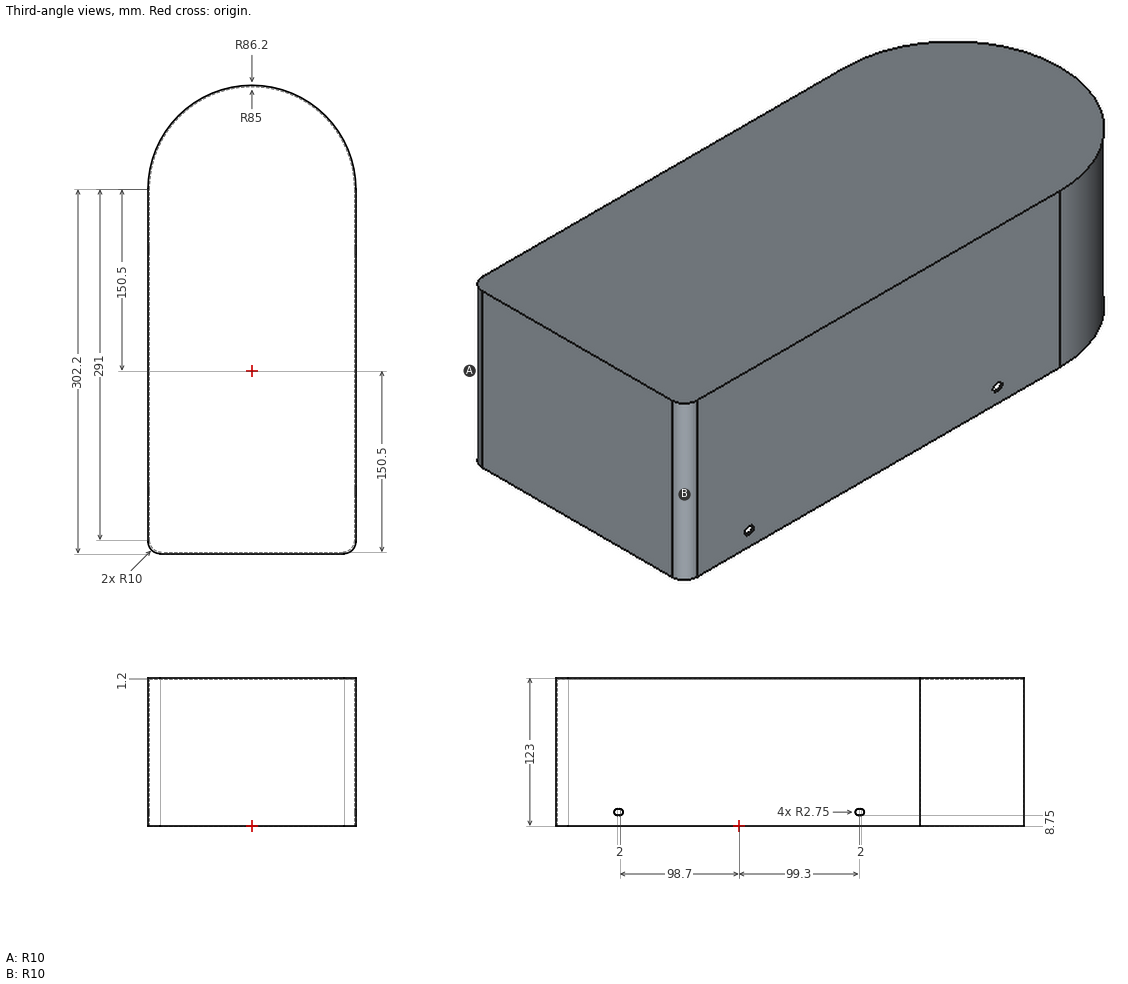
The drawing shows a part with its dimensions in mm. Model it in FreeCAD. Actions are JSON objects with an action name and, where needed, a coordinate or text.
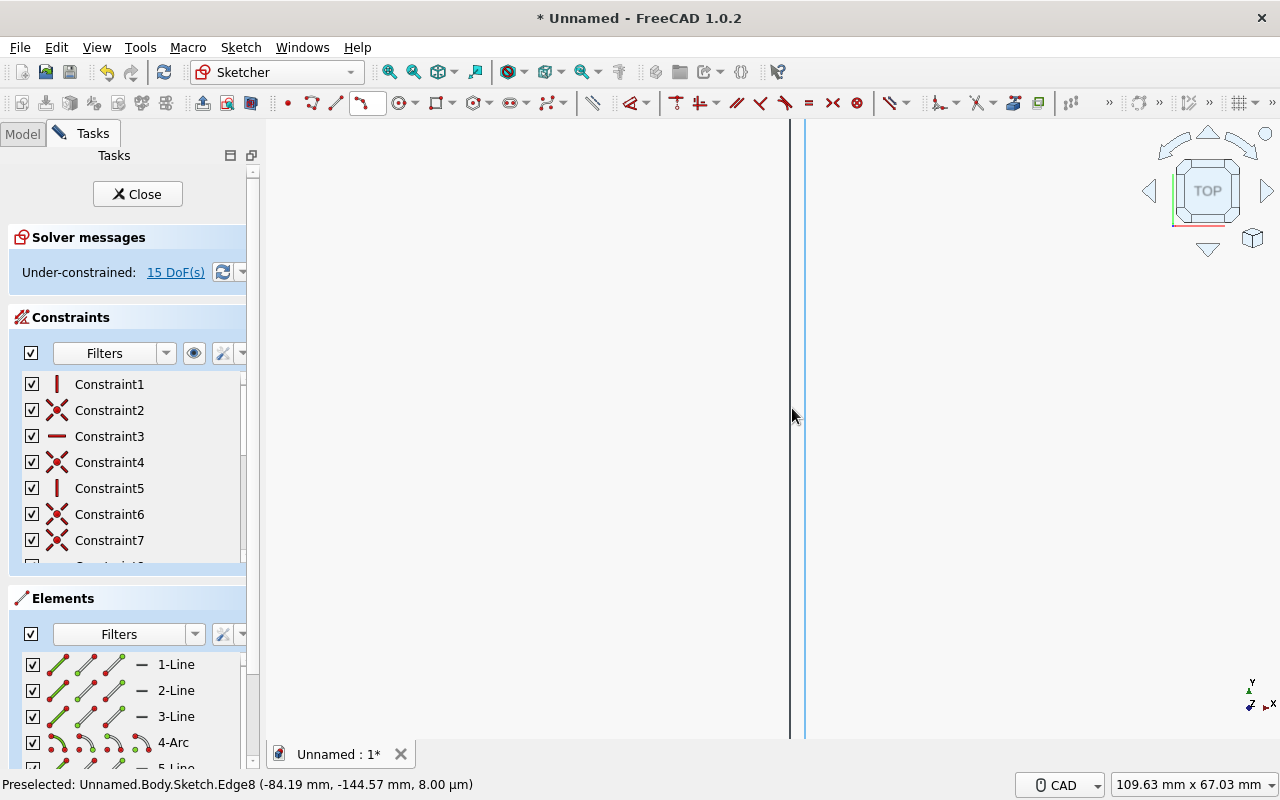
{"action": "left_click", "coordinate": [790, 405]}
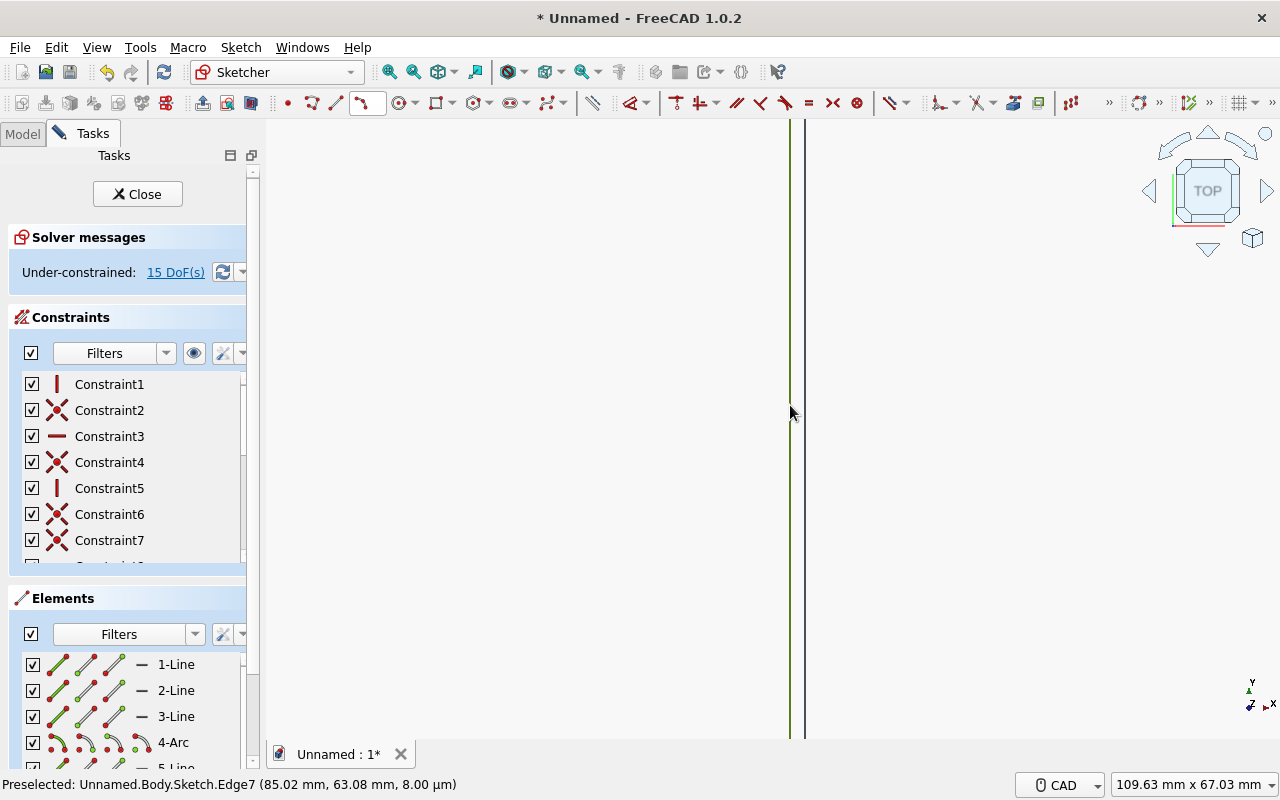
{"action": "scroll", "coordinate": [792, 408], "scroll_direction": "down", "scroll_amount": 11}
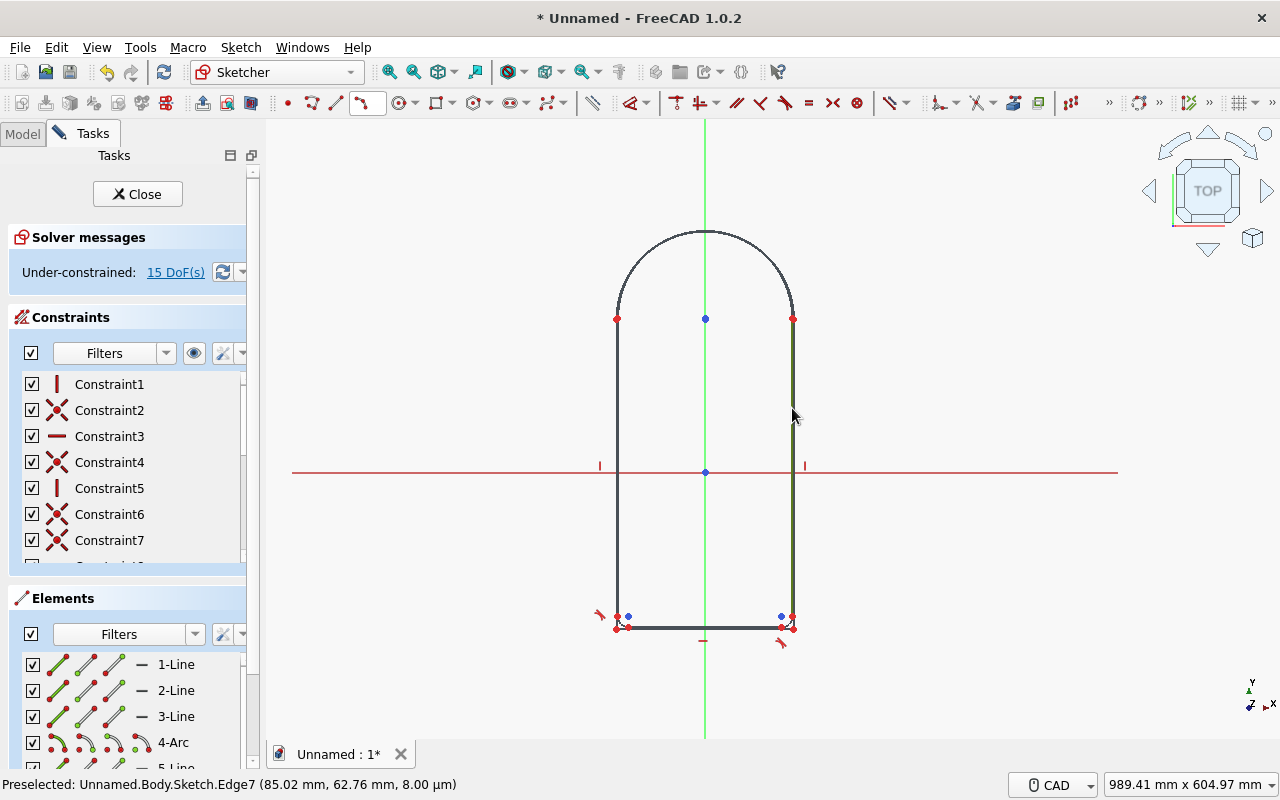
{"action": "scroll", "coordinate": [787, 626], "scroll_direction": "up", "scroll_amount": 8}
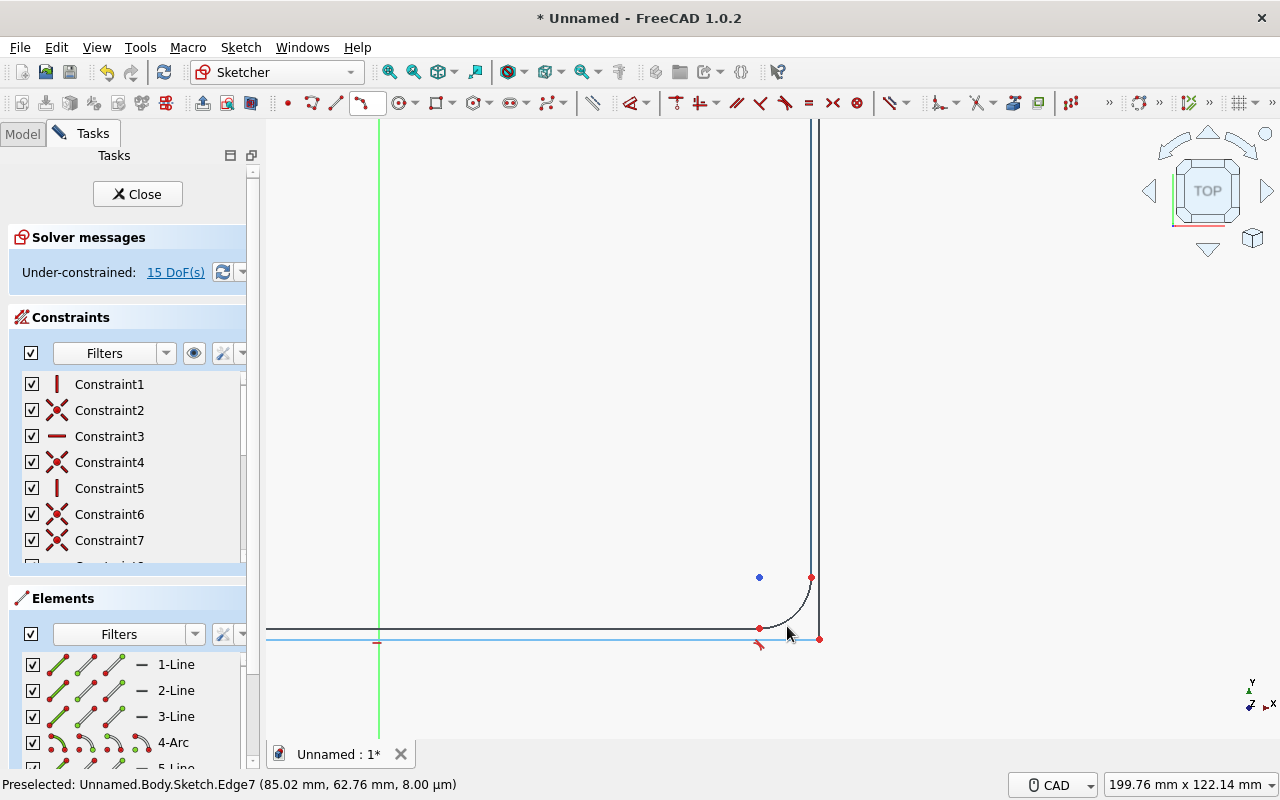
{"action": "left_click", "coordinate": [783, 623]}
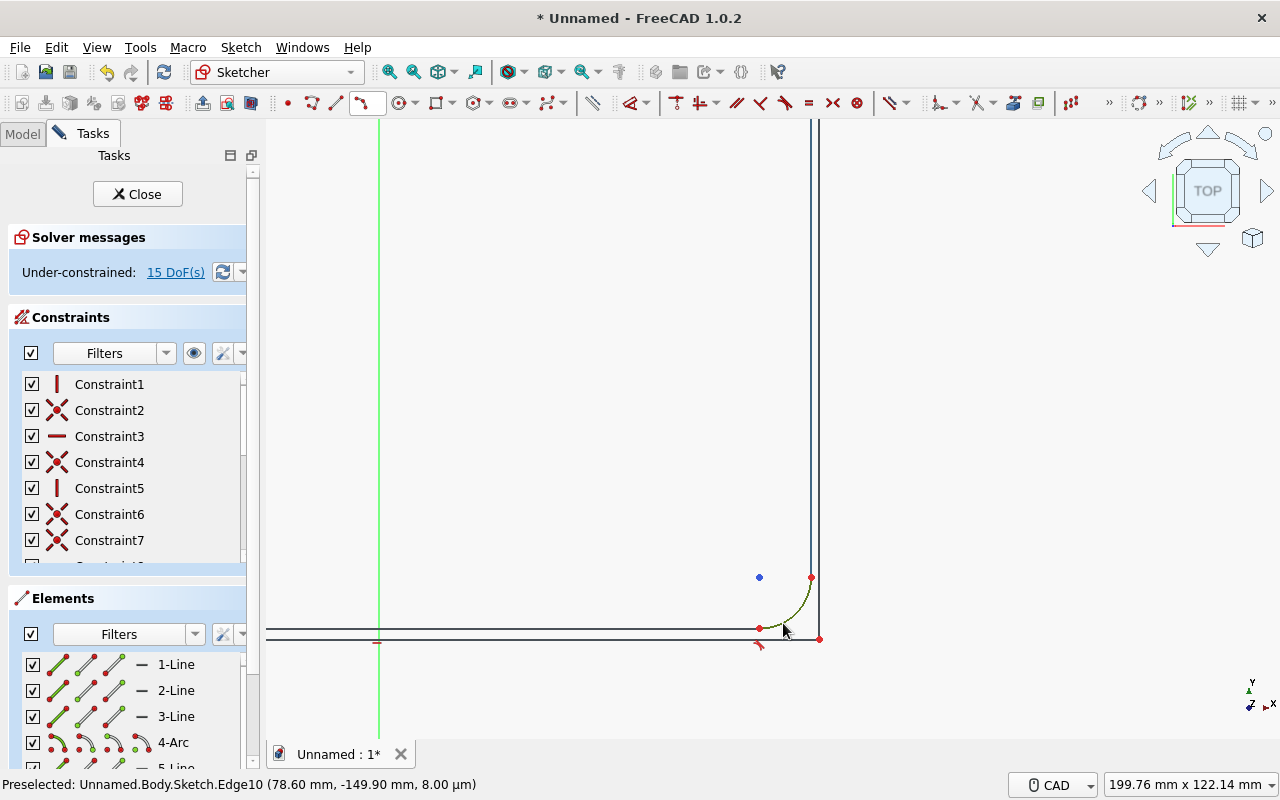
{"action": "left_click", "coordinate": [786, 104]}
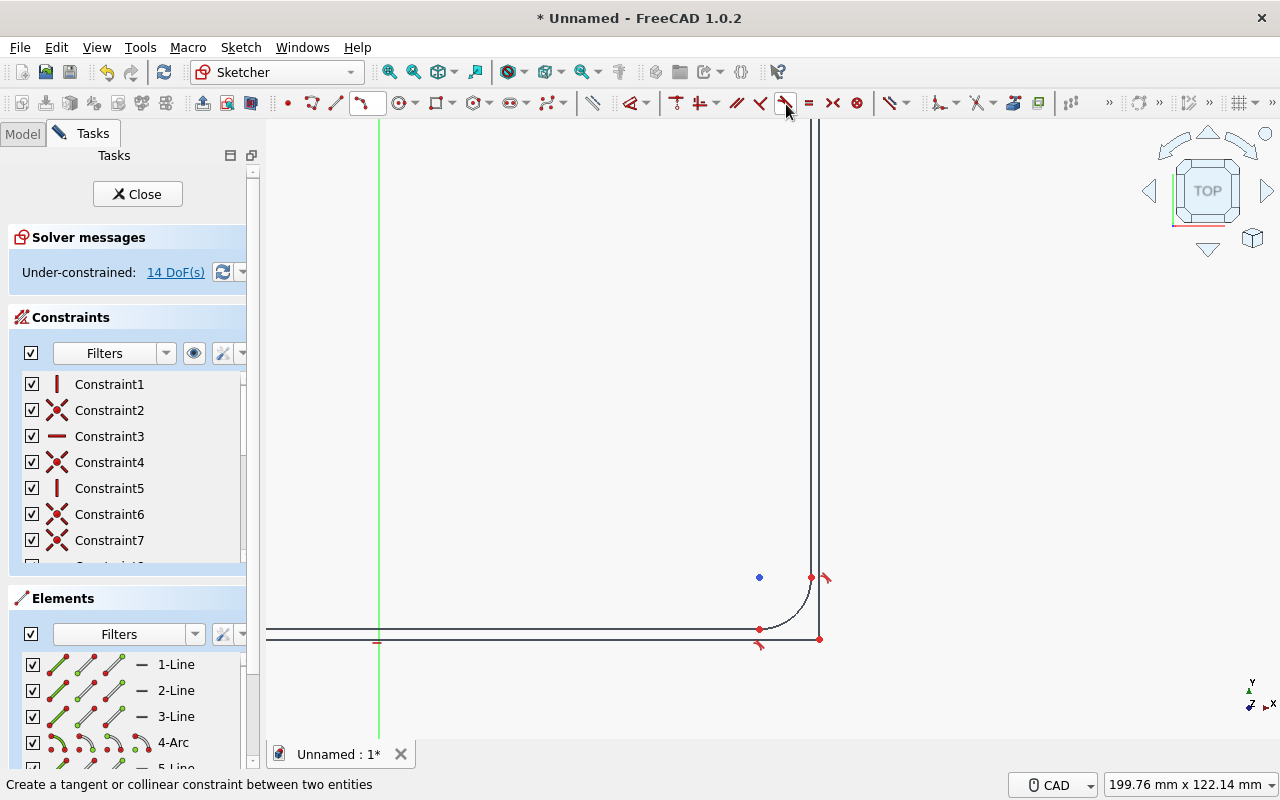
{"action": "scroll", "coordinate": [787, 626], "scroll_direction": "down", "scroll_amount": 8}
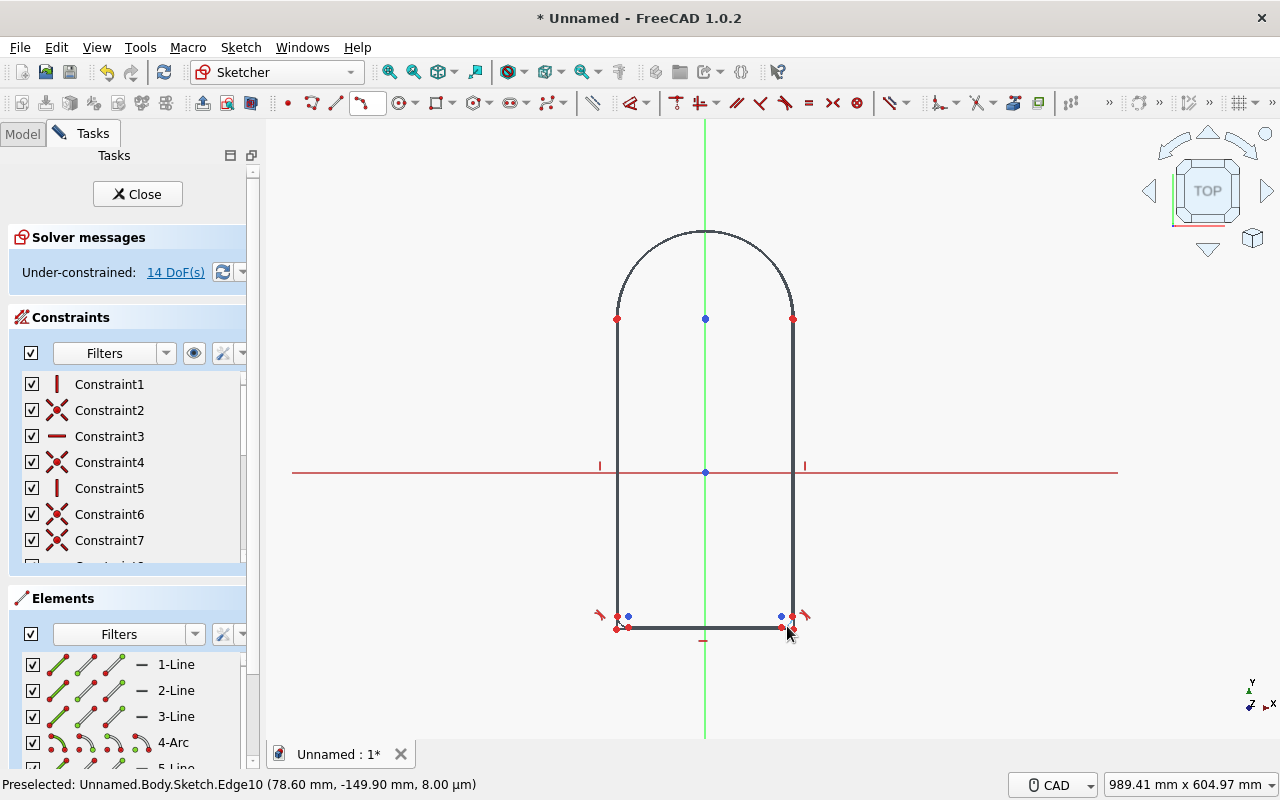
{"action": "scroll", "coordinate": [777, 267], "scroll_direction": "up", "scroll_amount": 13}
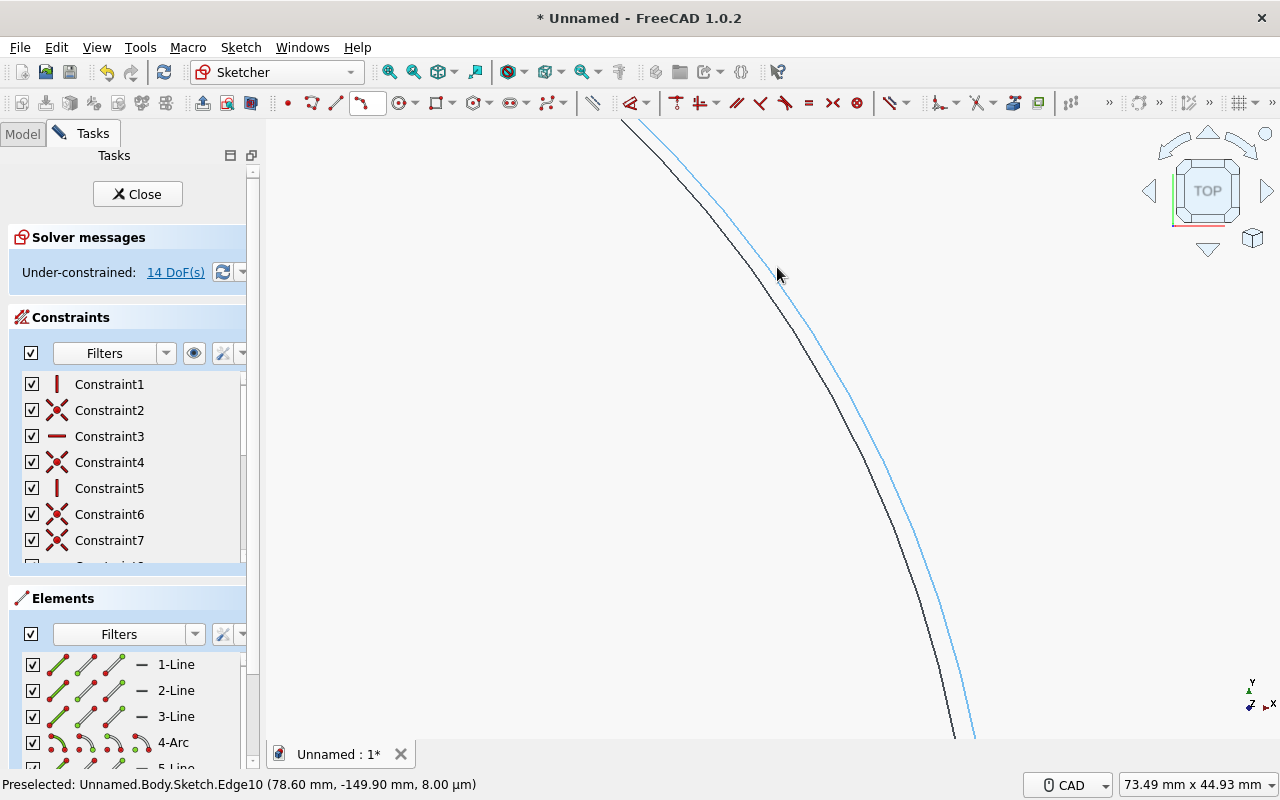
{"action": "left_click", "coordinate": [770, 270]}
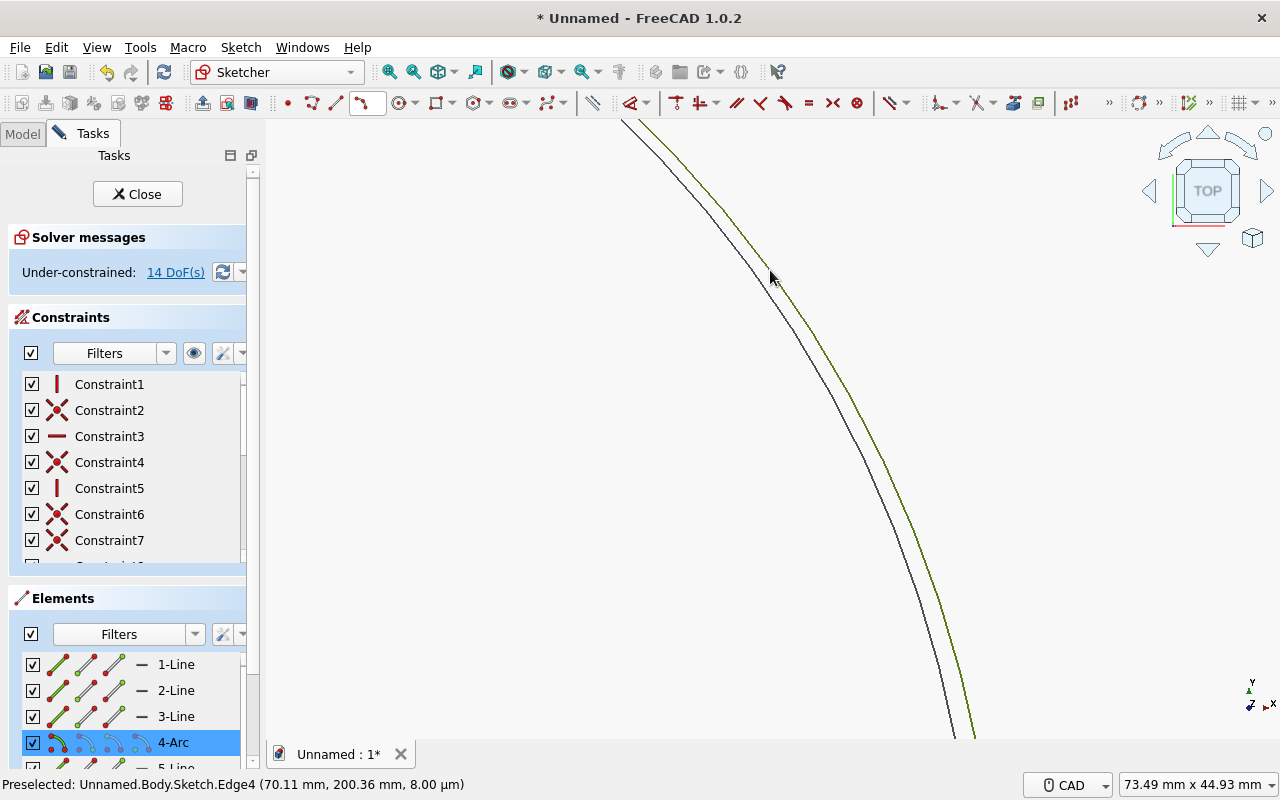
{"action": "left_click", "coordinate": [752, 269]}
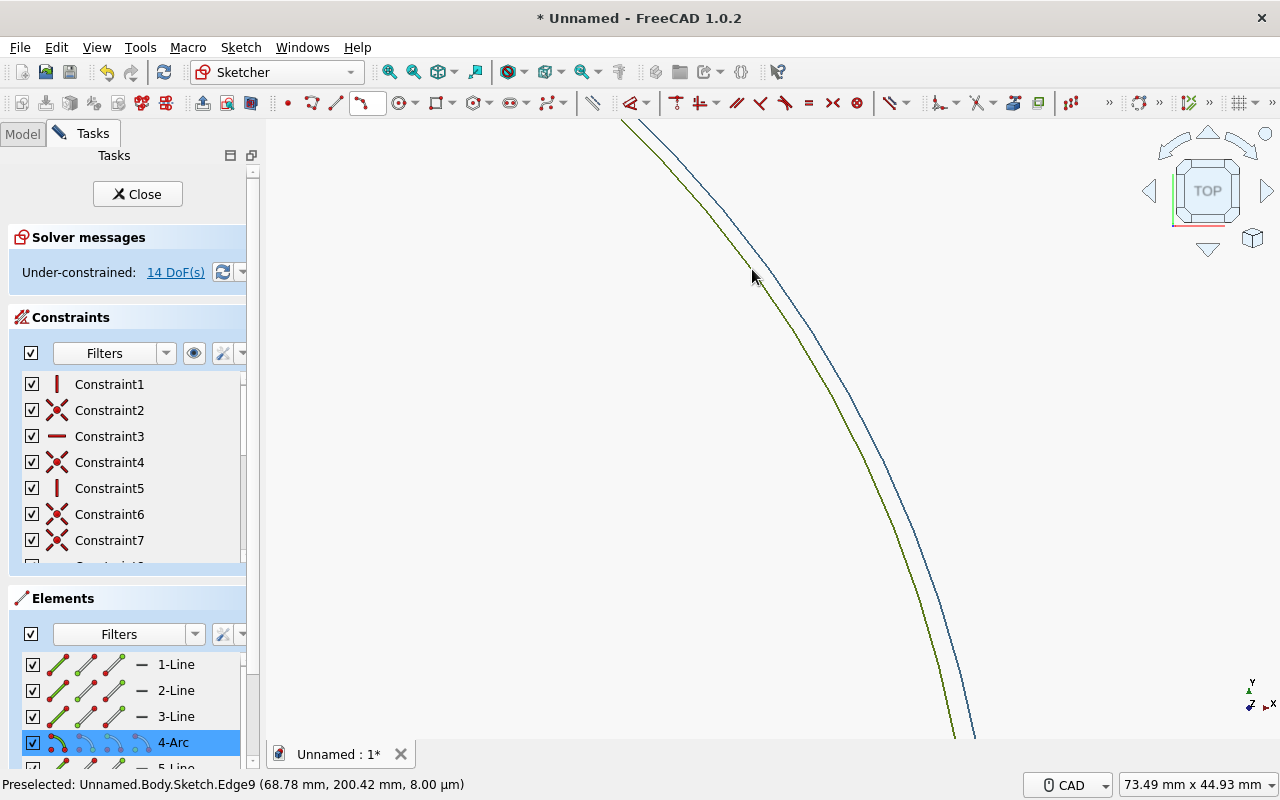
{"action": "key", "text": "c"}